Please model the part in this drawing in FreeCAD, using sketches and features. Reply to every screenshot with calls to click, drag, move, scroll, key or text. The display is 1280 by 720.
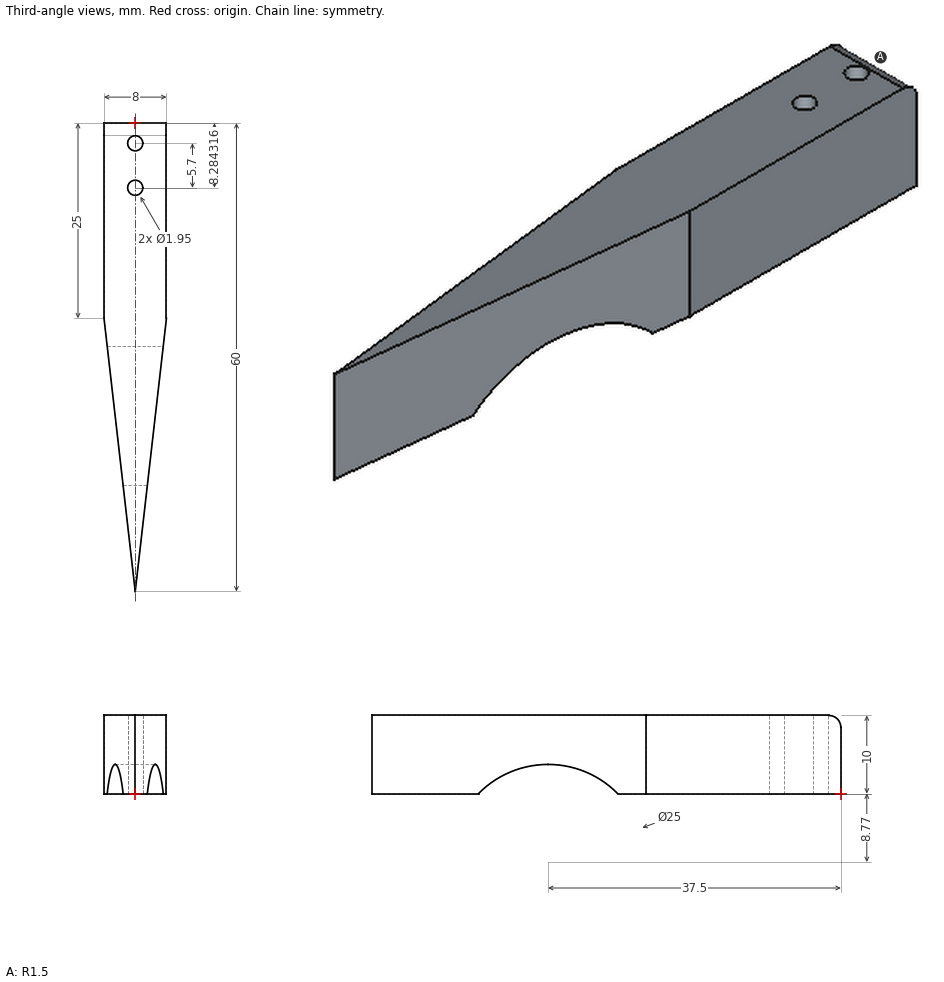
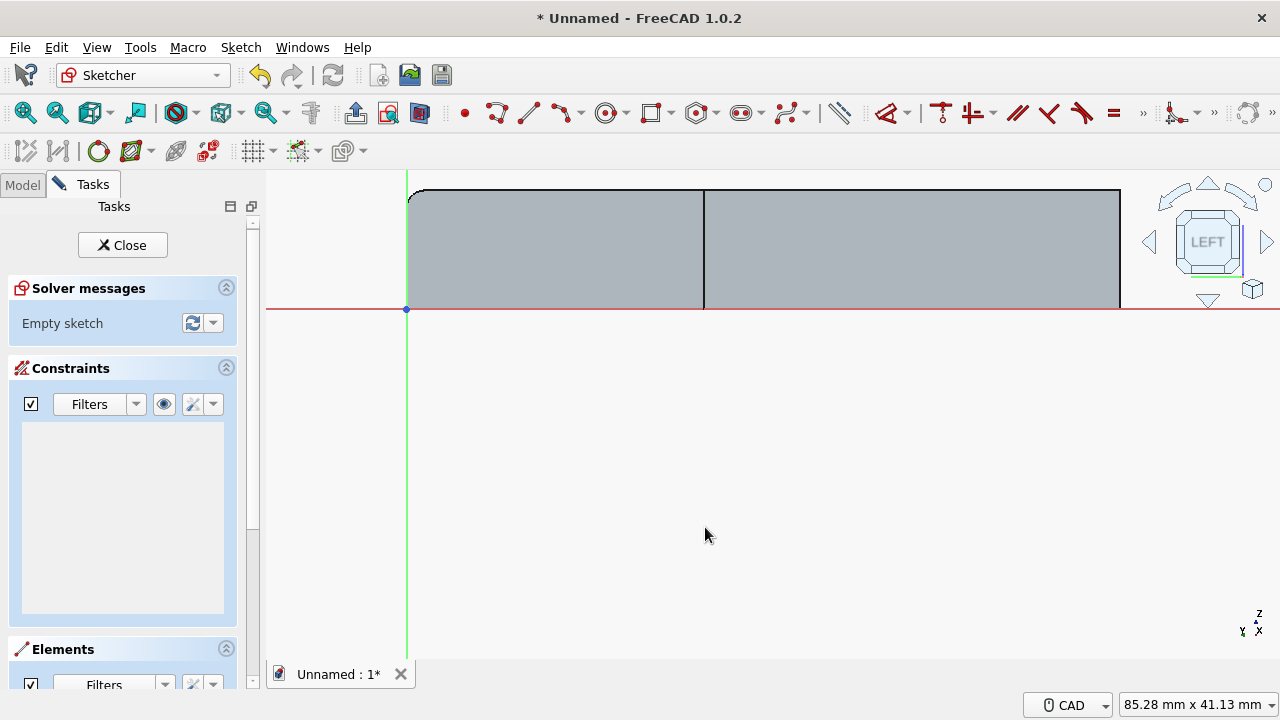
key(g)
key(c)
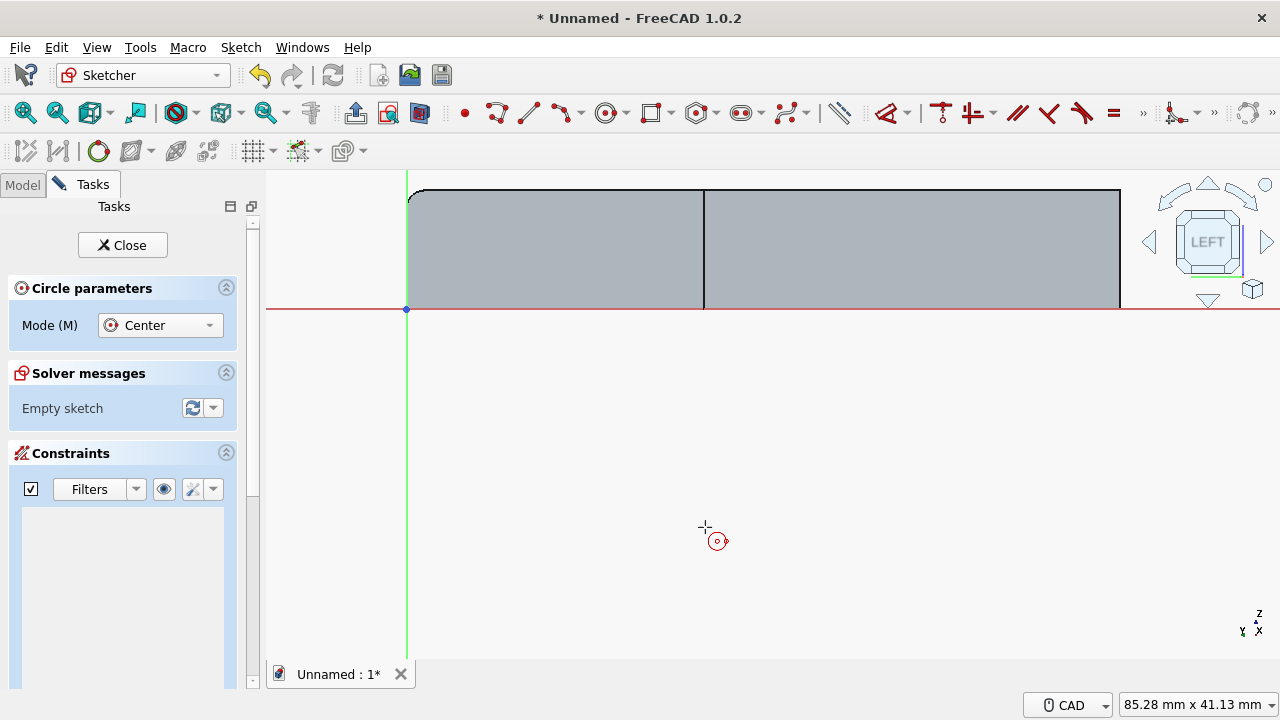
click(852, 414)
move(958, 519)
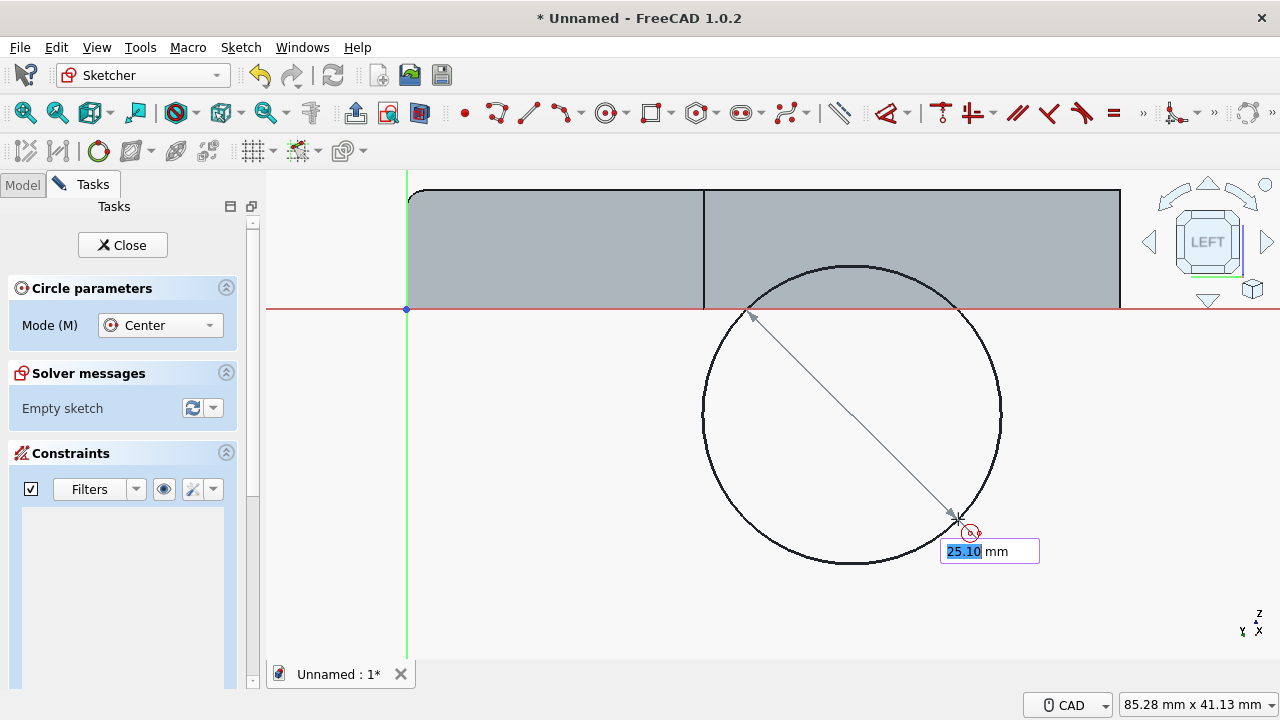
text(25)
key(Return)
key(Escape)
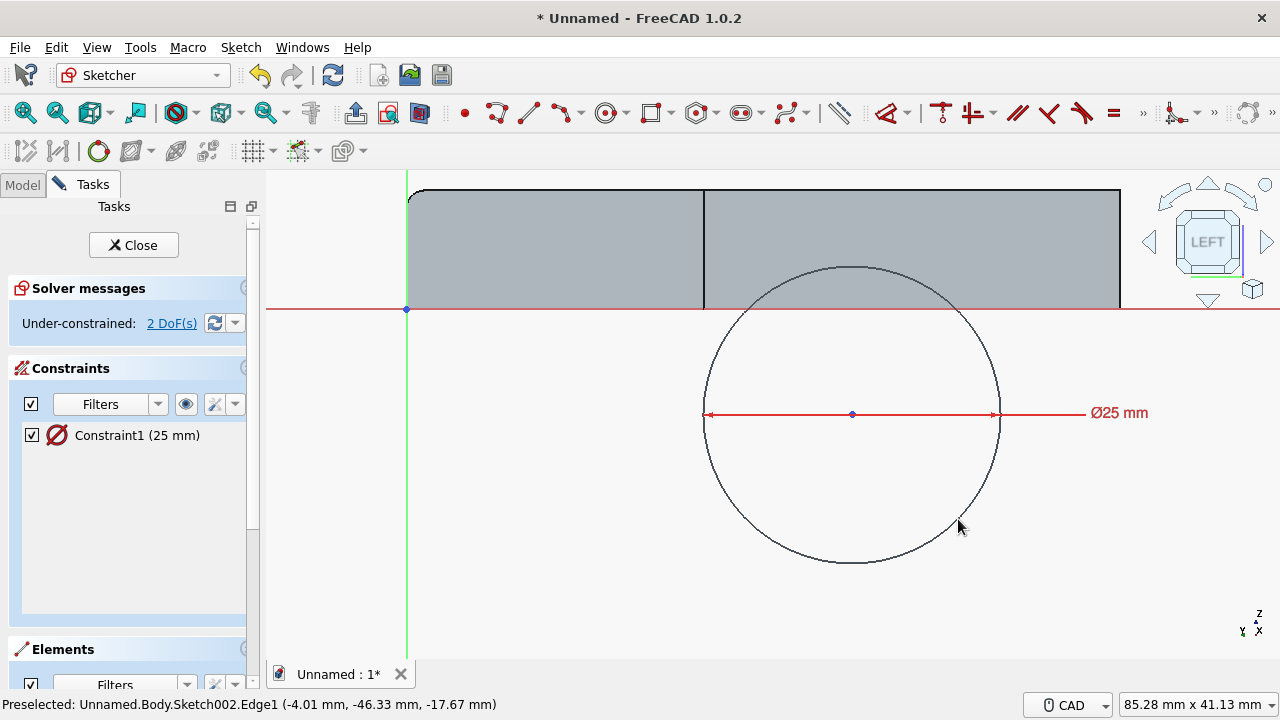
key(d)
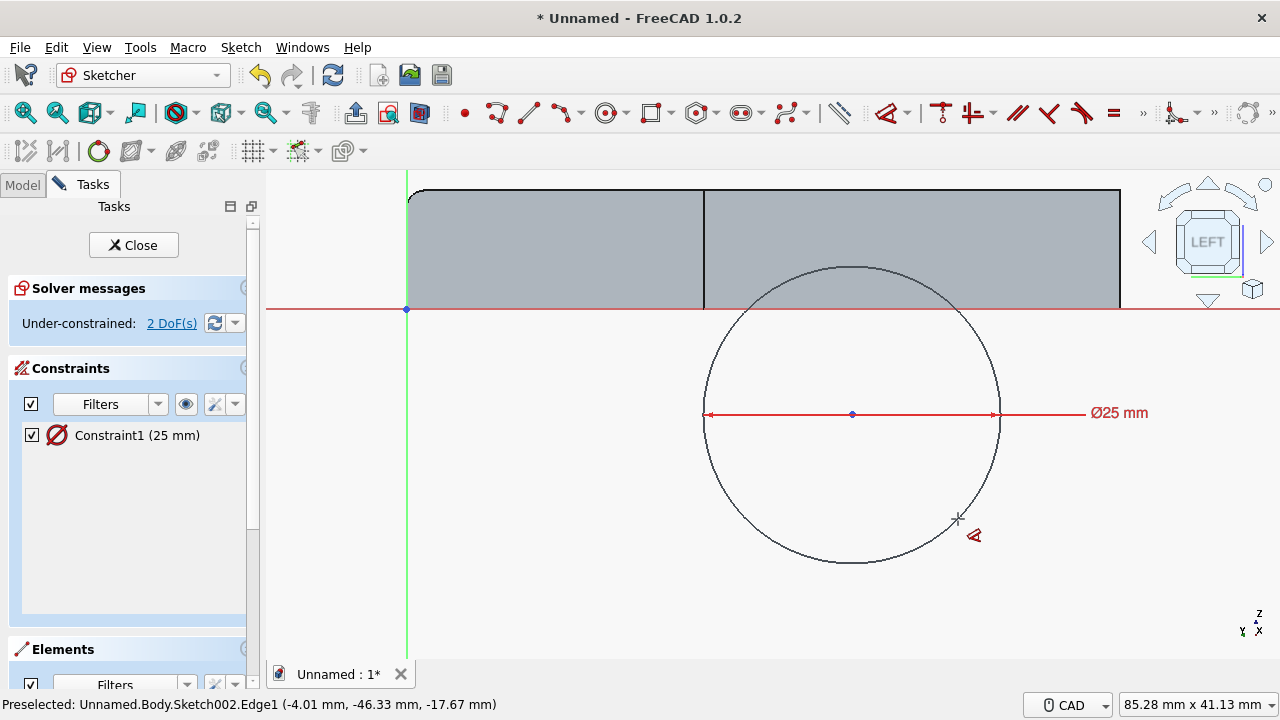
click(852, 415)
click(629, 275)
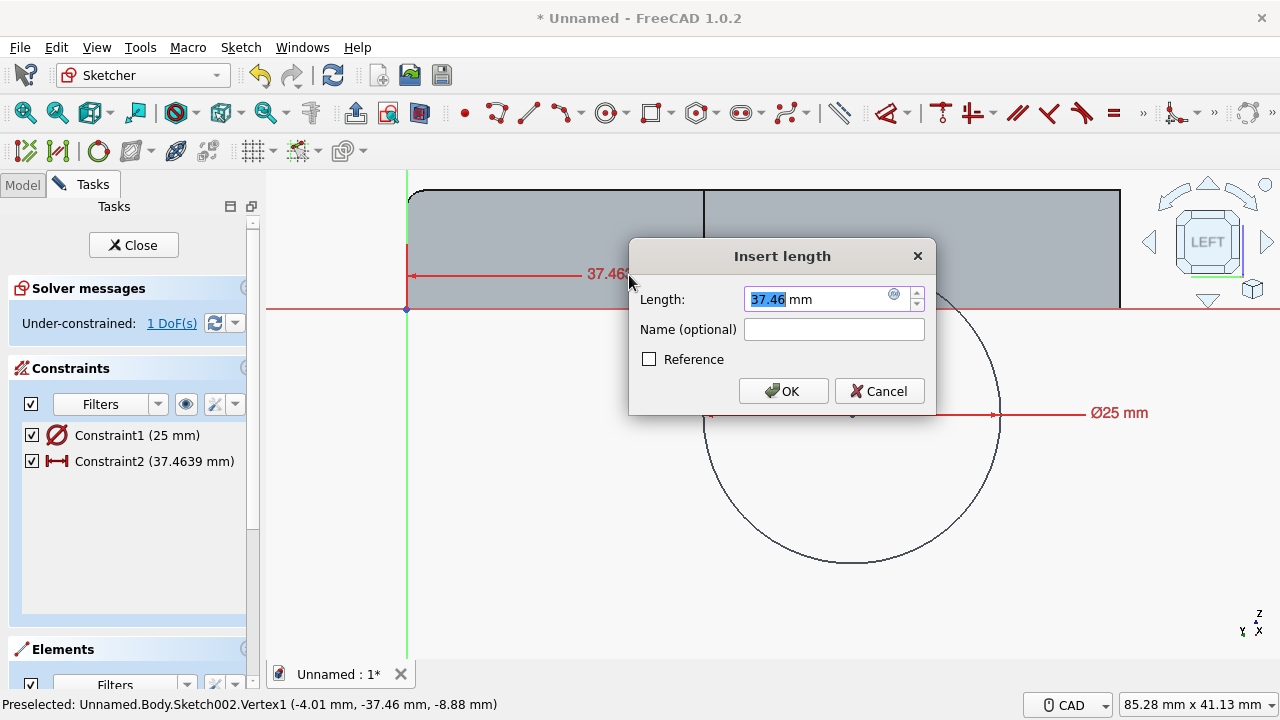
text(37.5)
key(Return)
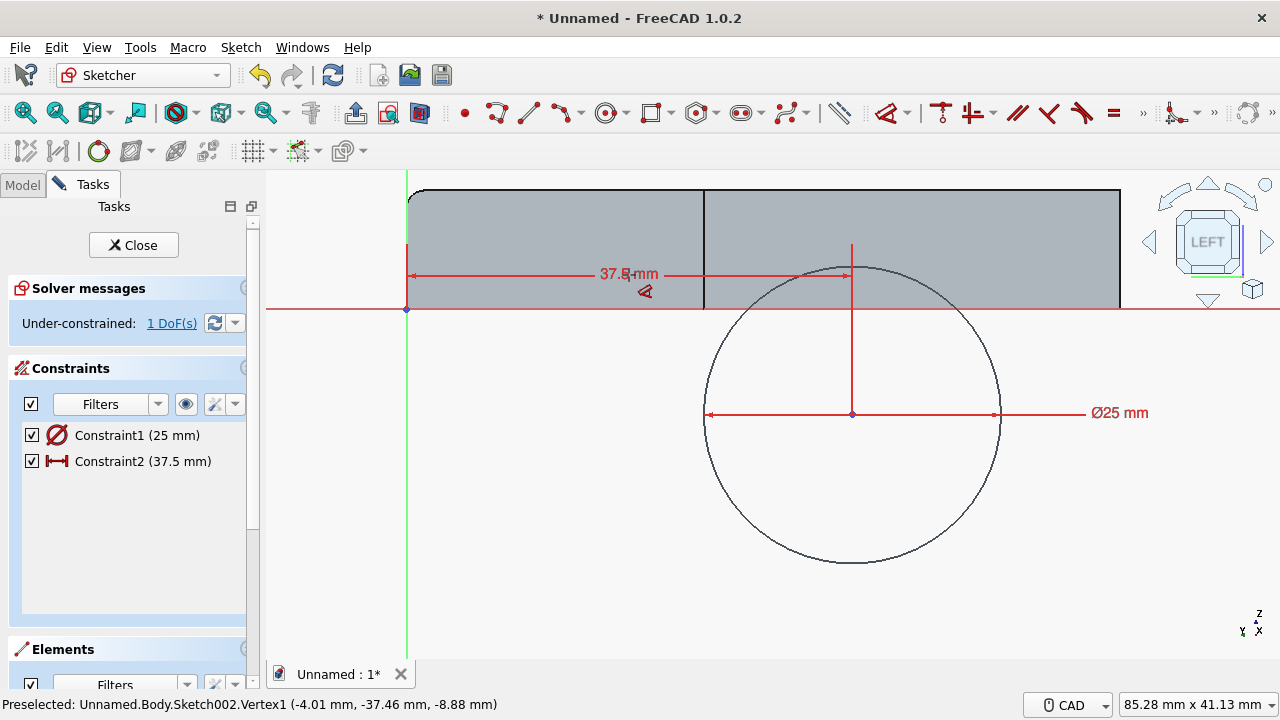
click(852, 415)
click(373, 362)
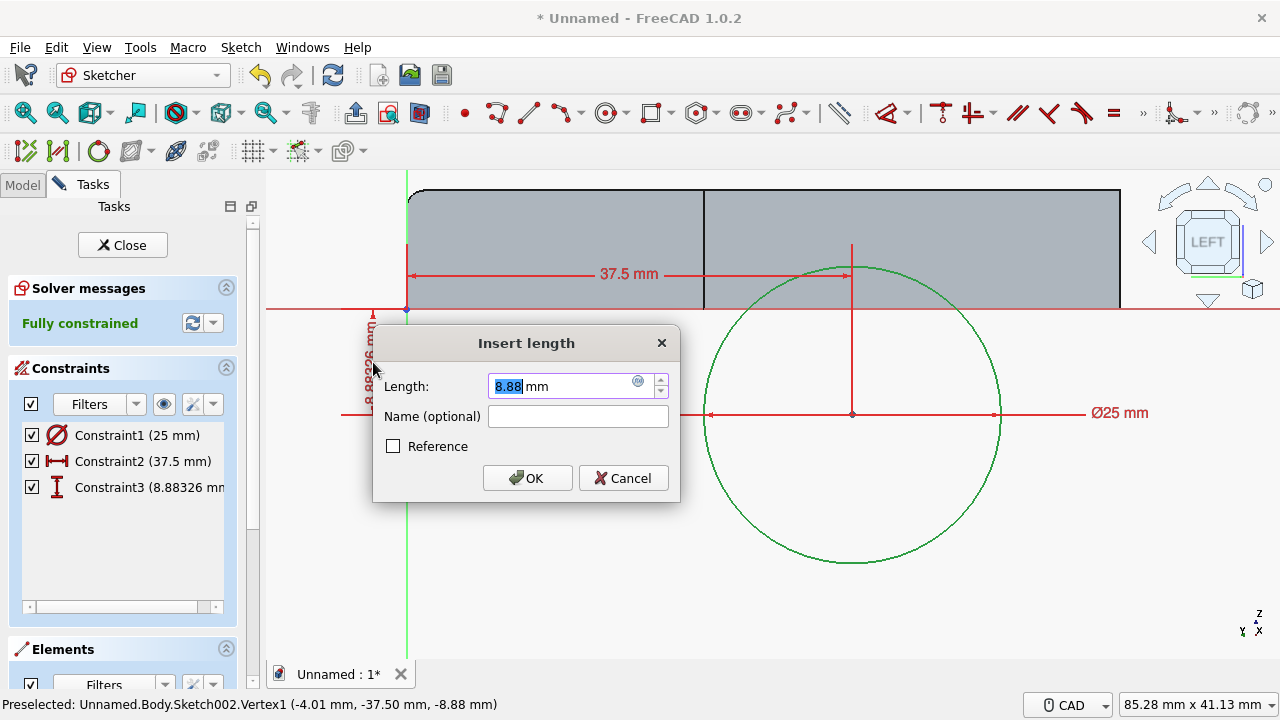
text(8.77)
key(Return)
key(Escape)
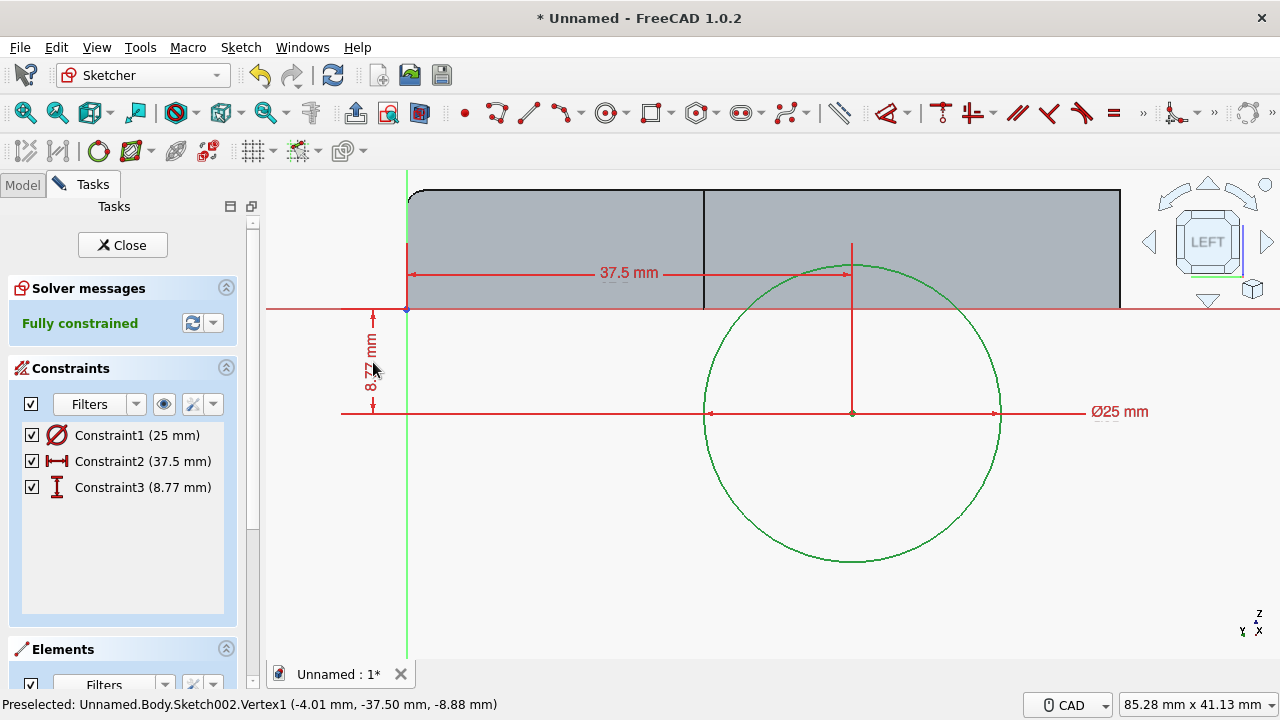
click(123, 245)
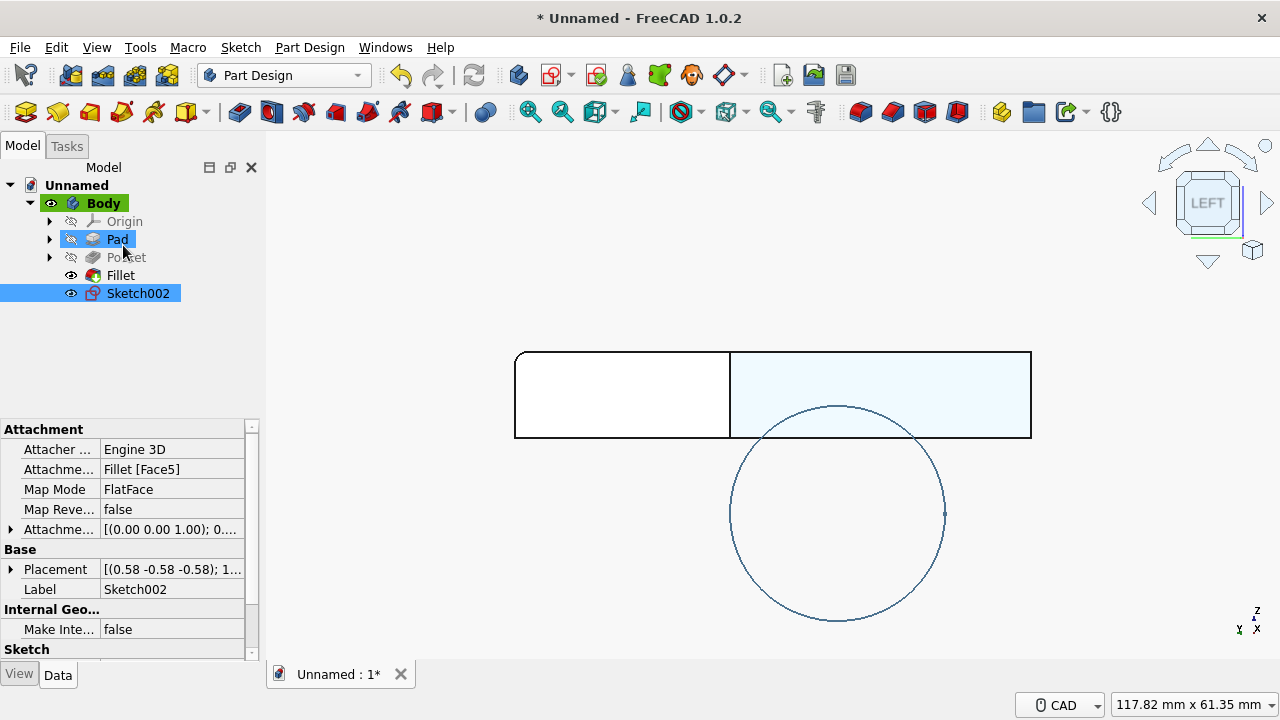
click(240, 112)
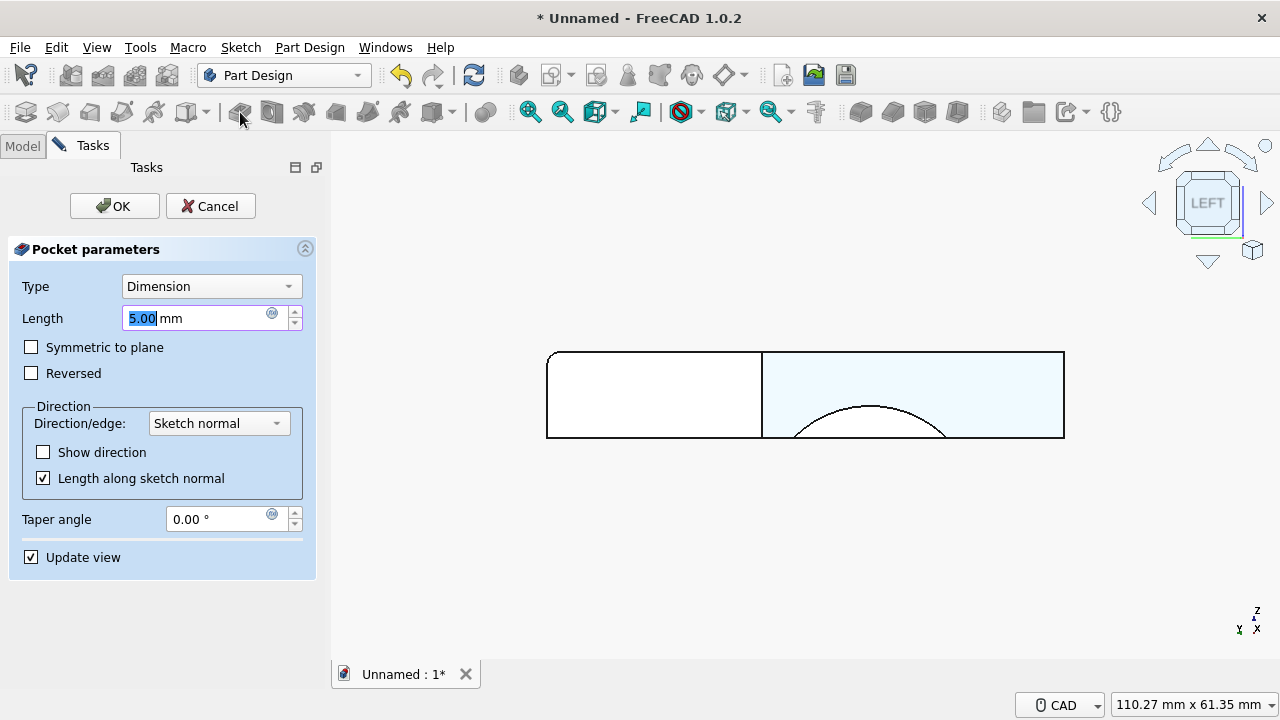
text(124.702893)
key(Tab)